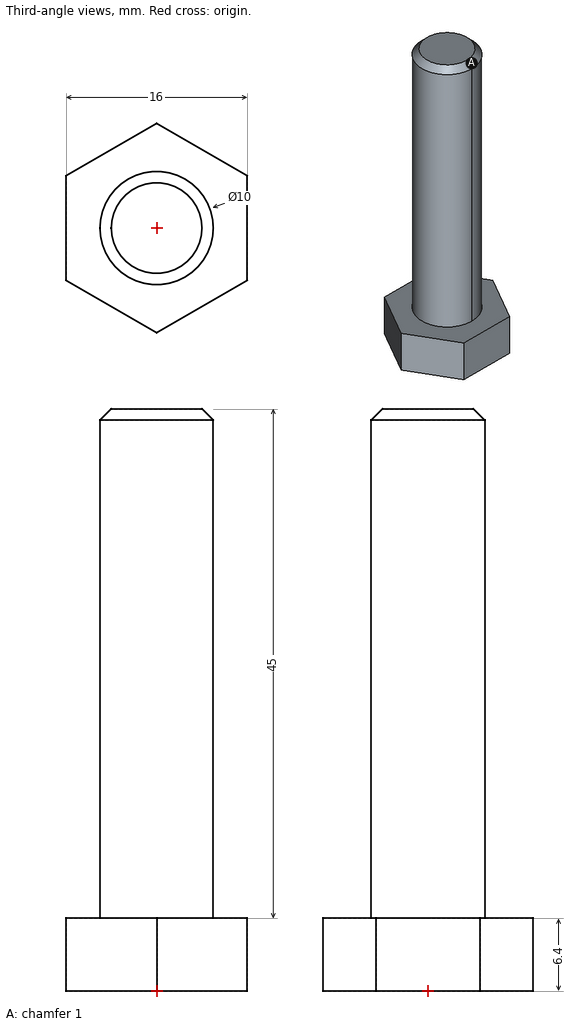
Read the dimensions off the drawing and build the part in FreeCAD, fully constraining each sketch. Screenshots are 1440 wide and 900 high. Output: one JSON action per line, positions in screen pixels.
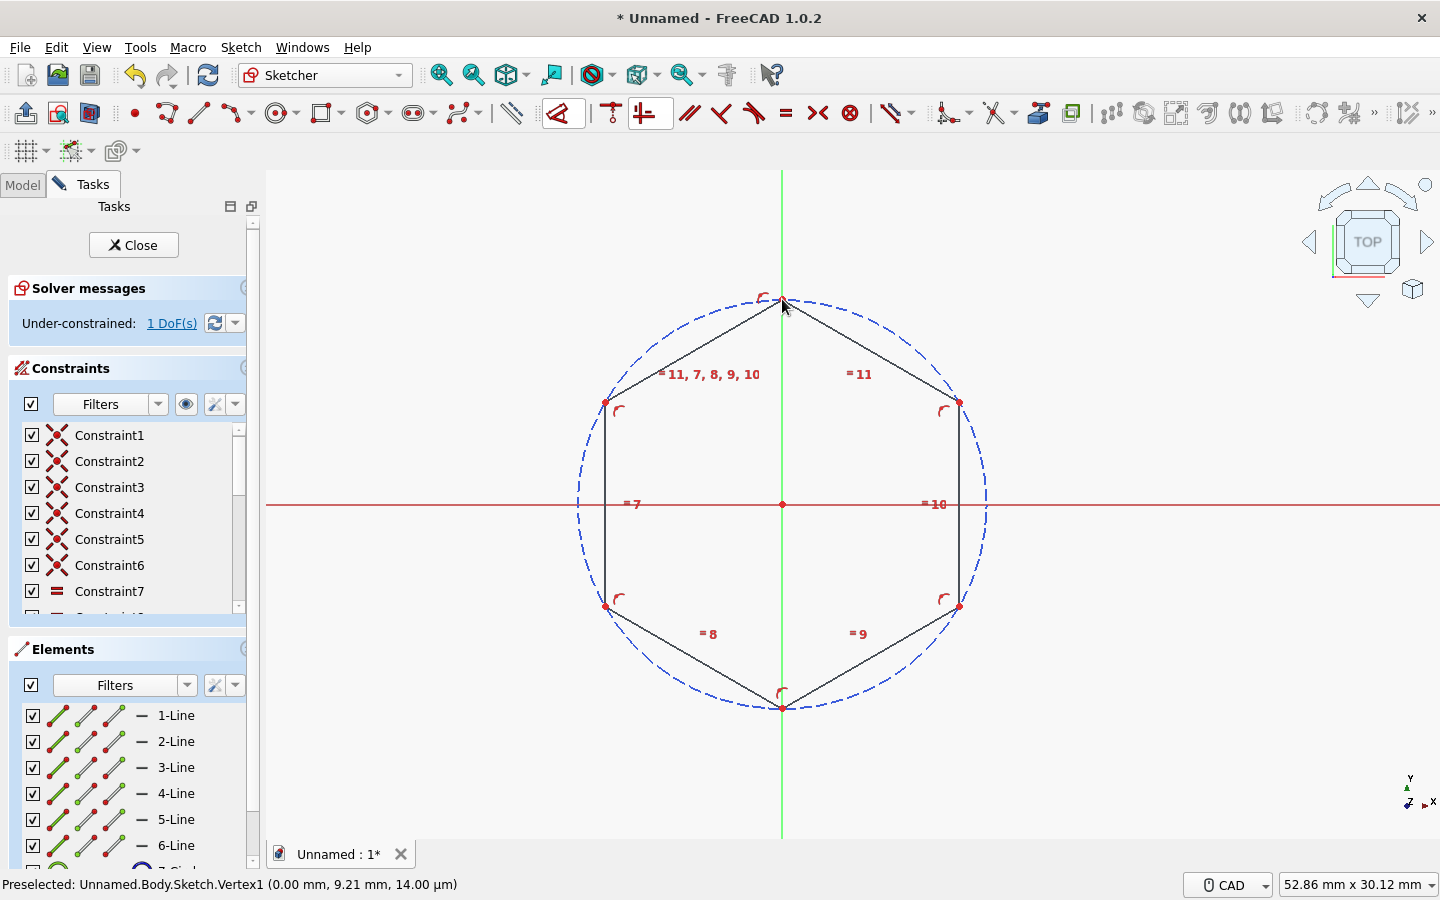
{"action": "left_click", "coordinate": [605, 402]}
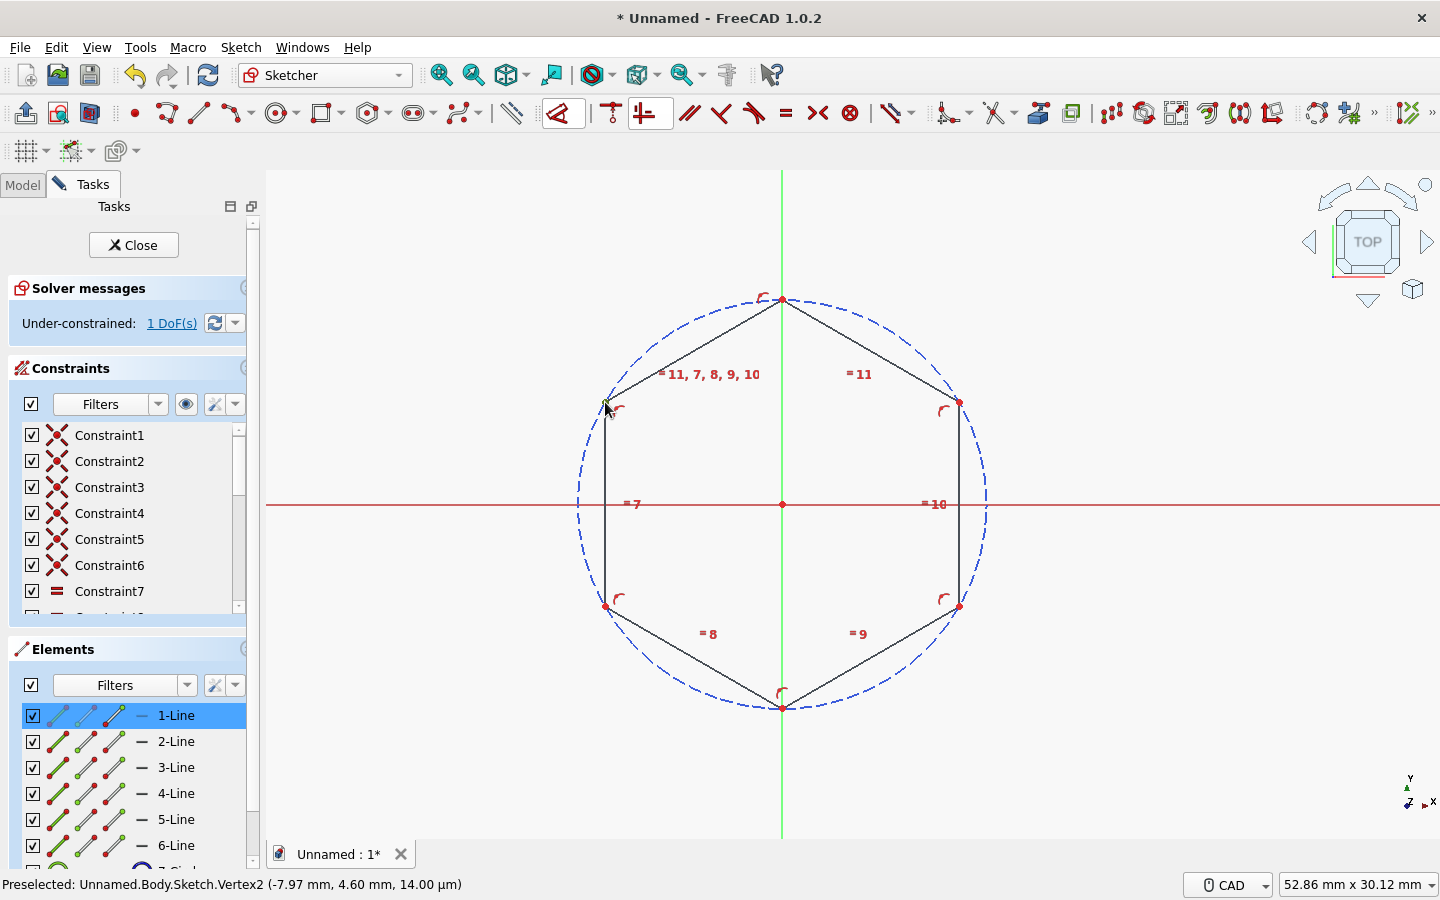
{"action": "left_click", "coordinate": [959, 607]}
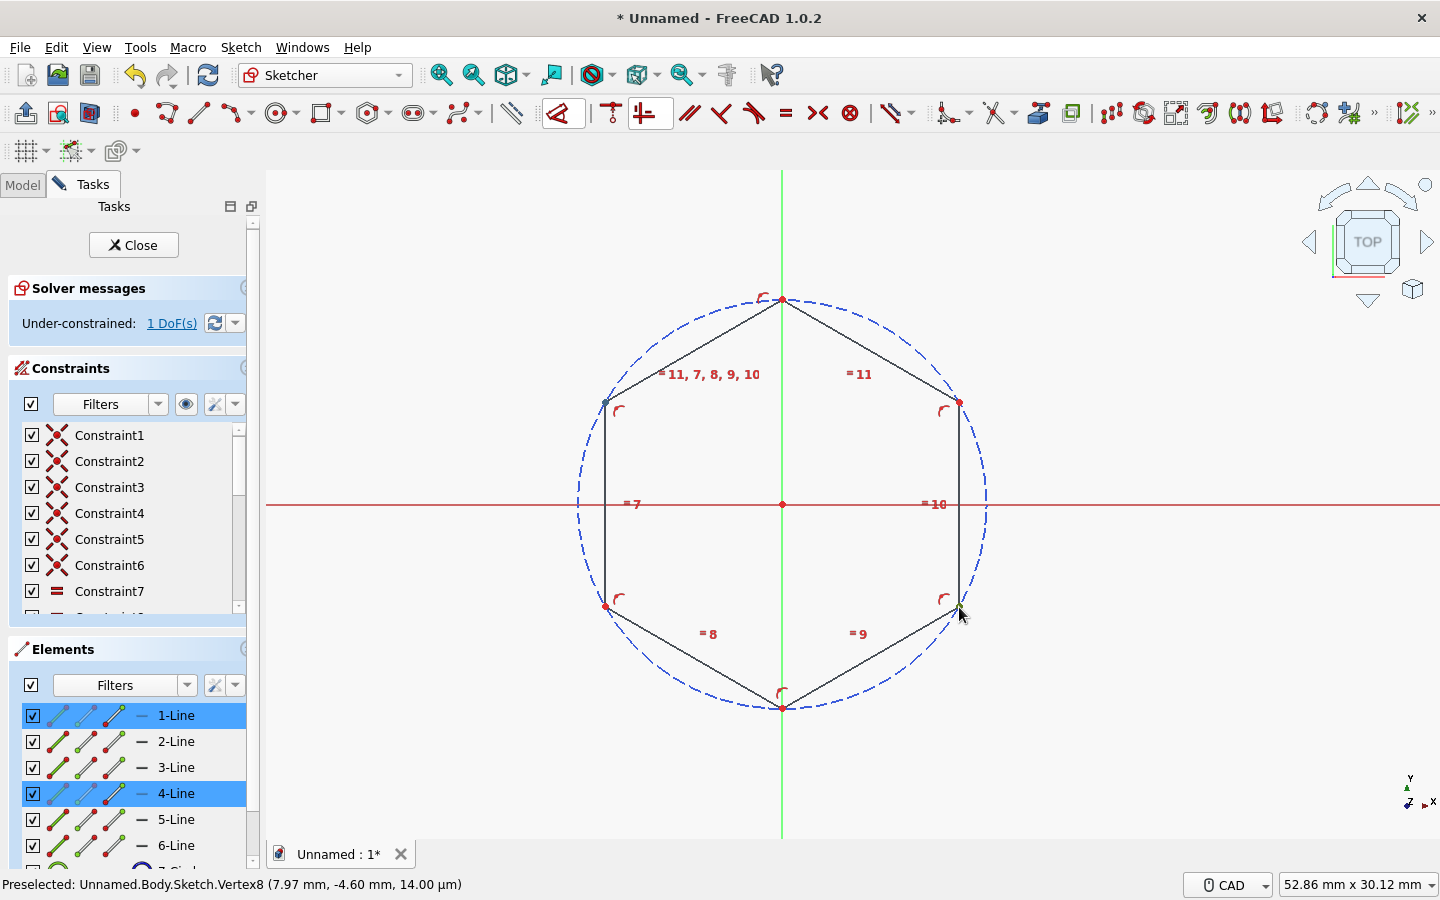
{"action": "left_click", "coordinate": [580, 114]}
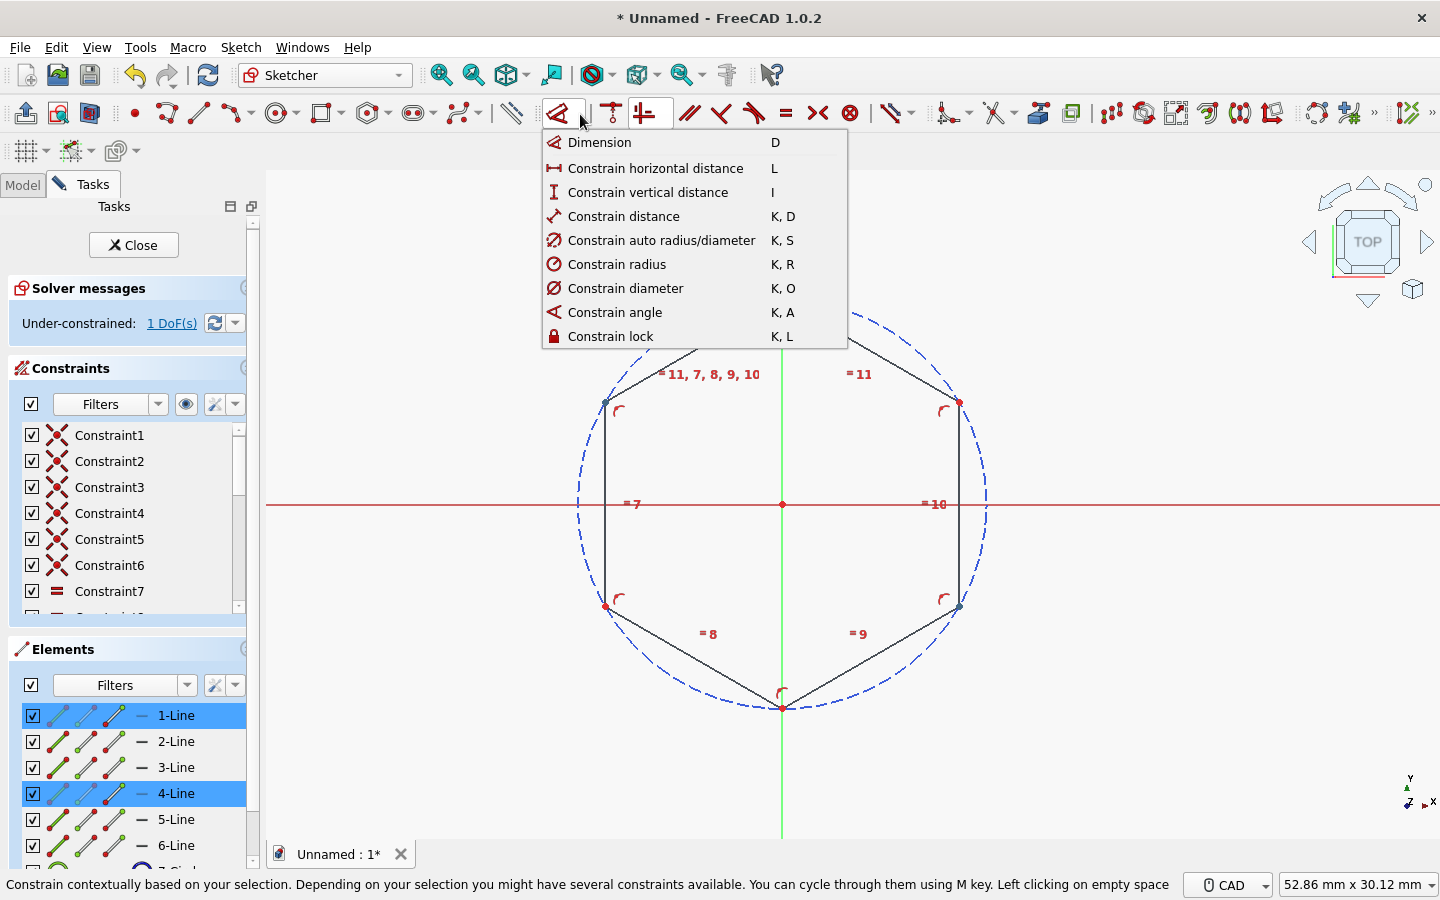
{"action": "left_click", "coordinate": [695, 168]}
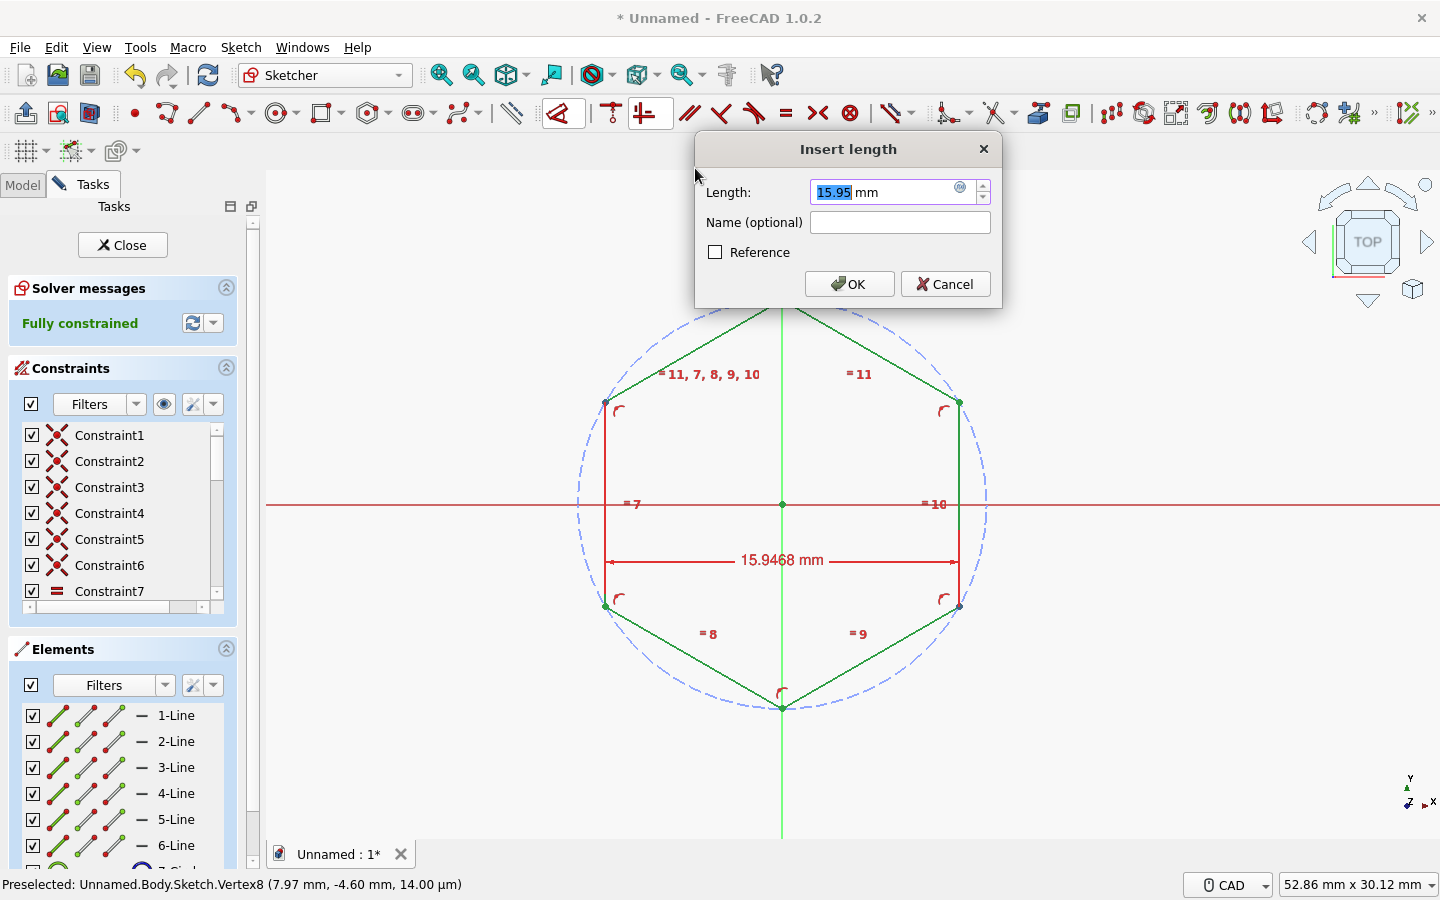
{"action": "type", "text": "16"}
{"action": "key", "text": "Return"}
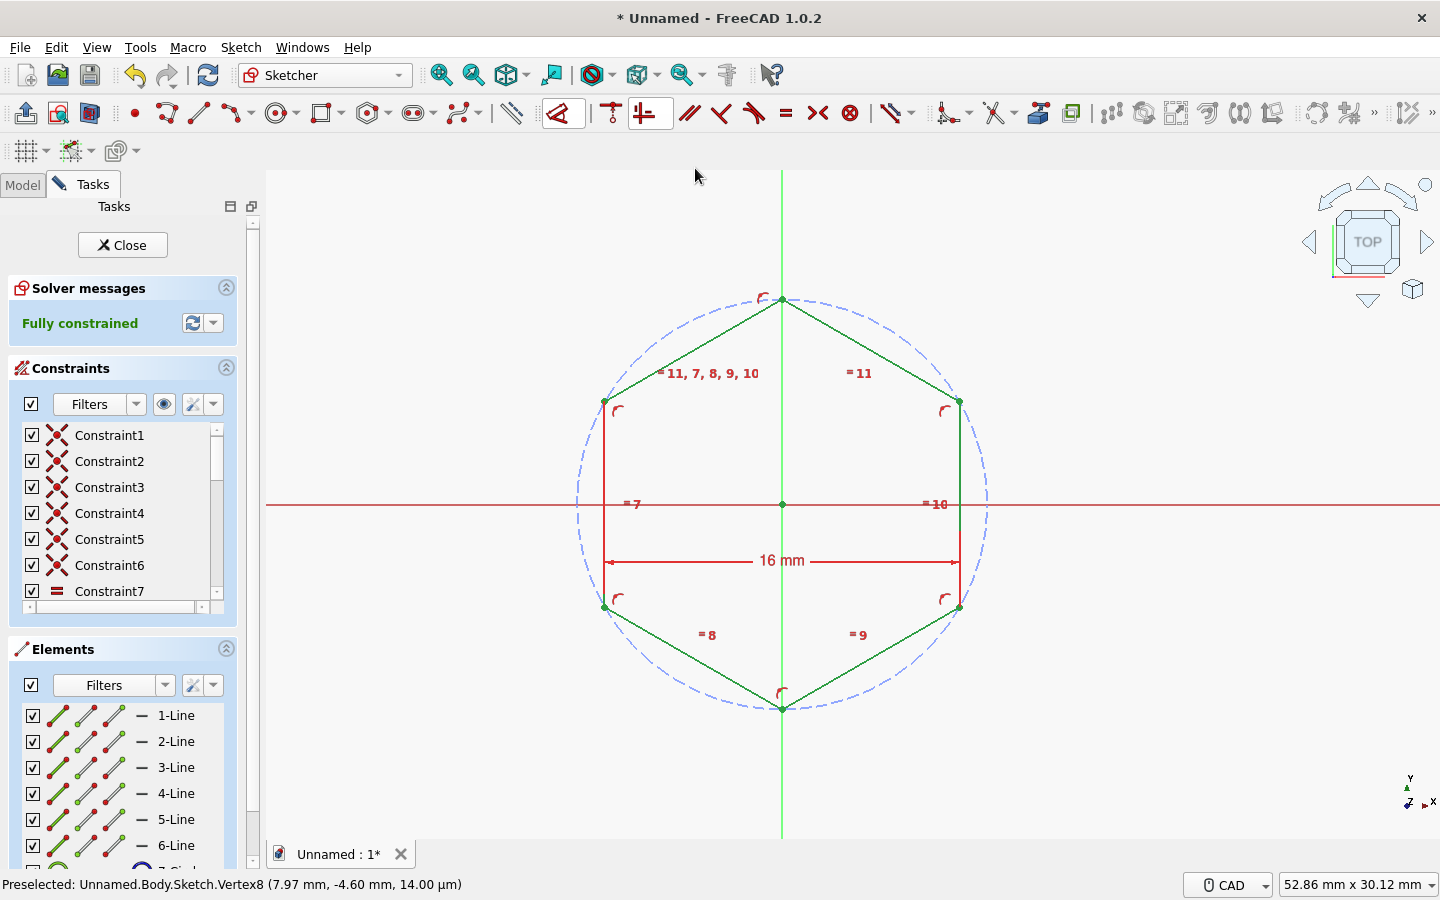
{"action": "left_click", "coordinate": [123, 245]}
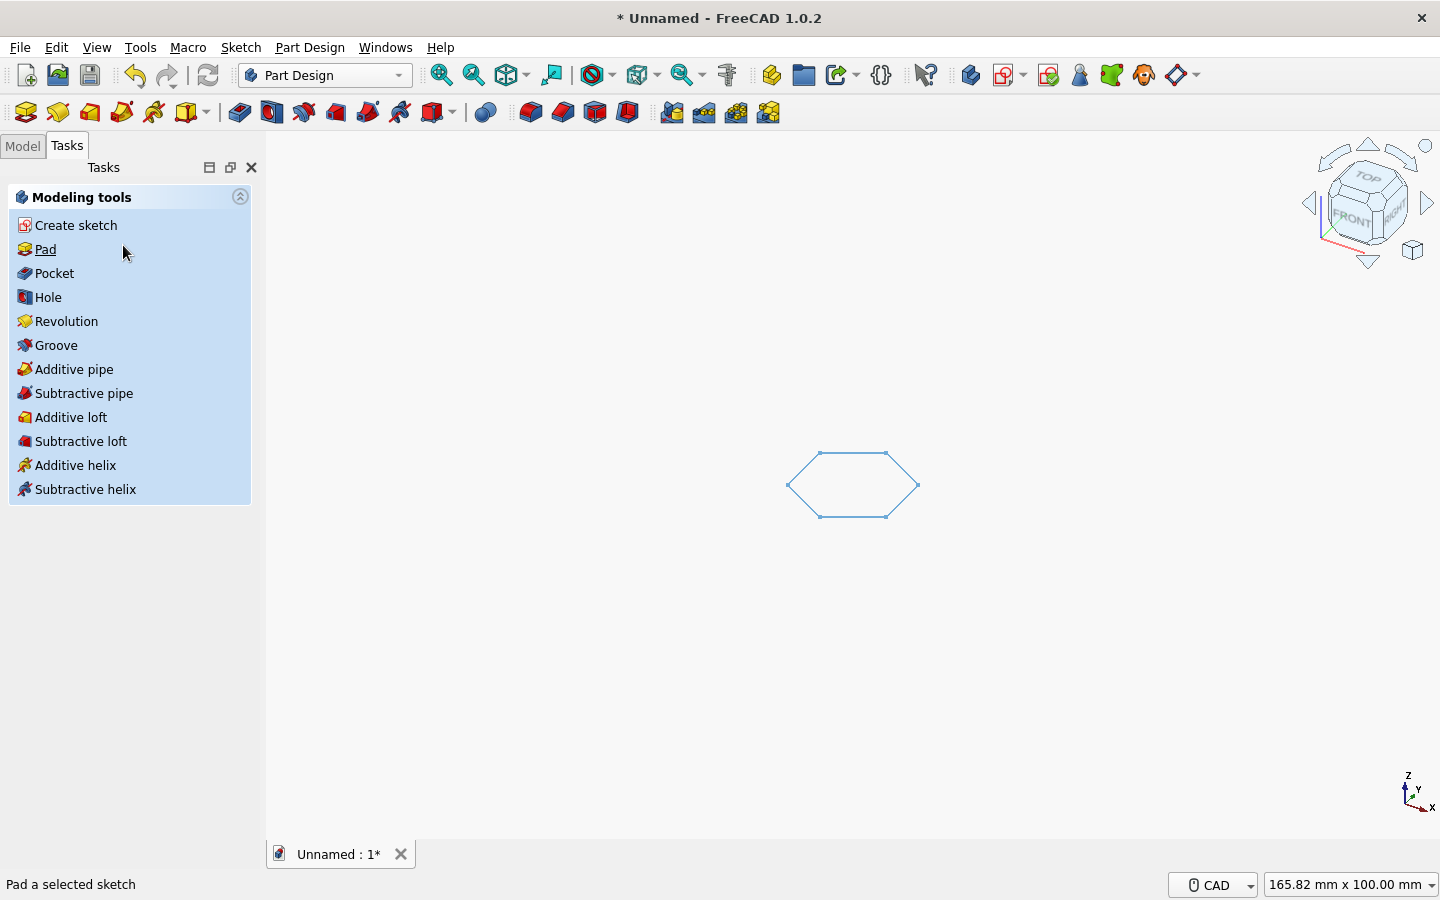
{"action": "left_click", "coordinate": [26, 112]}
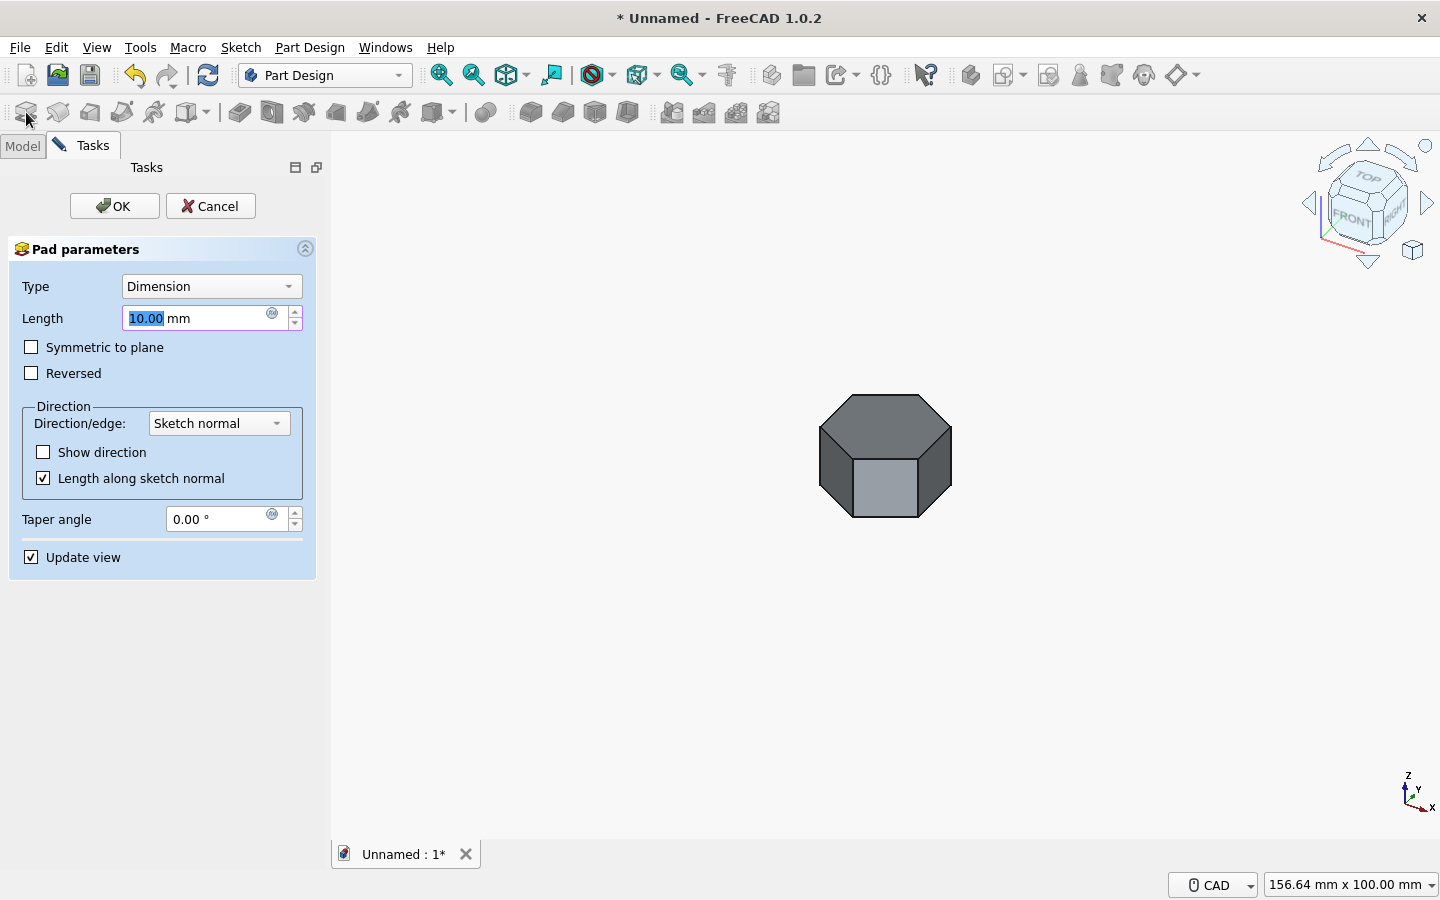
{"action": "type", "text": "6.4"}
{"action": "key", "text": "Tab"}